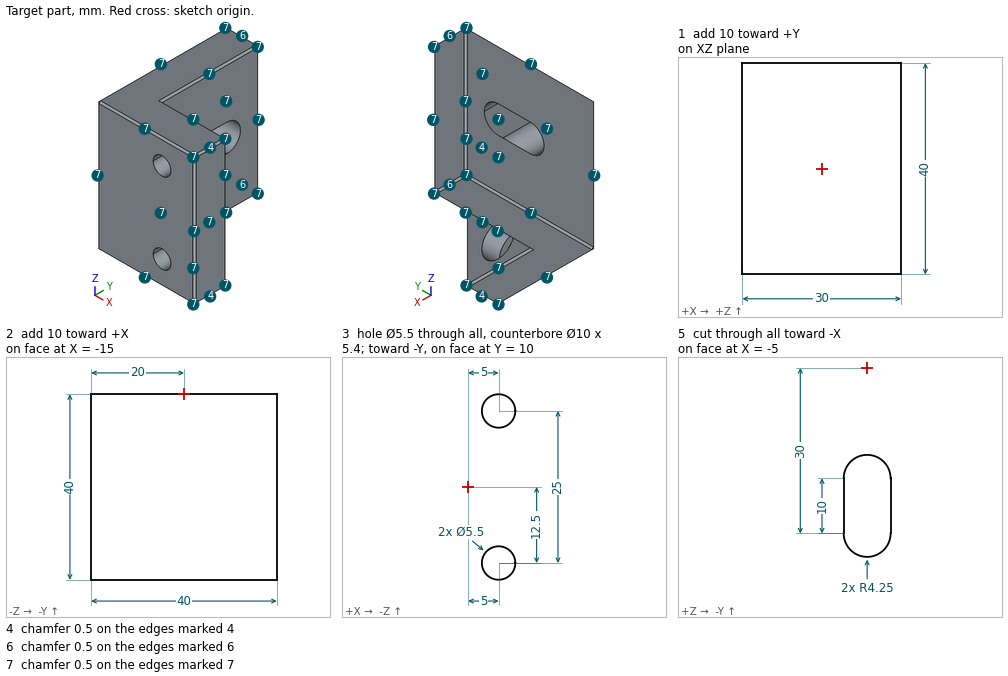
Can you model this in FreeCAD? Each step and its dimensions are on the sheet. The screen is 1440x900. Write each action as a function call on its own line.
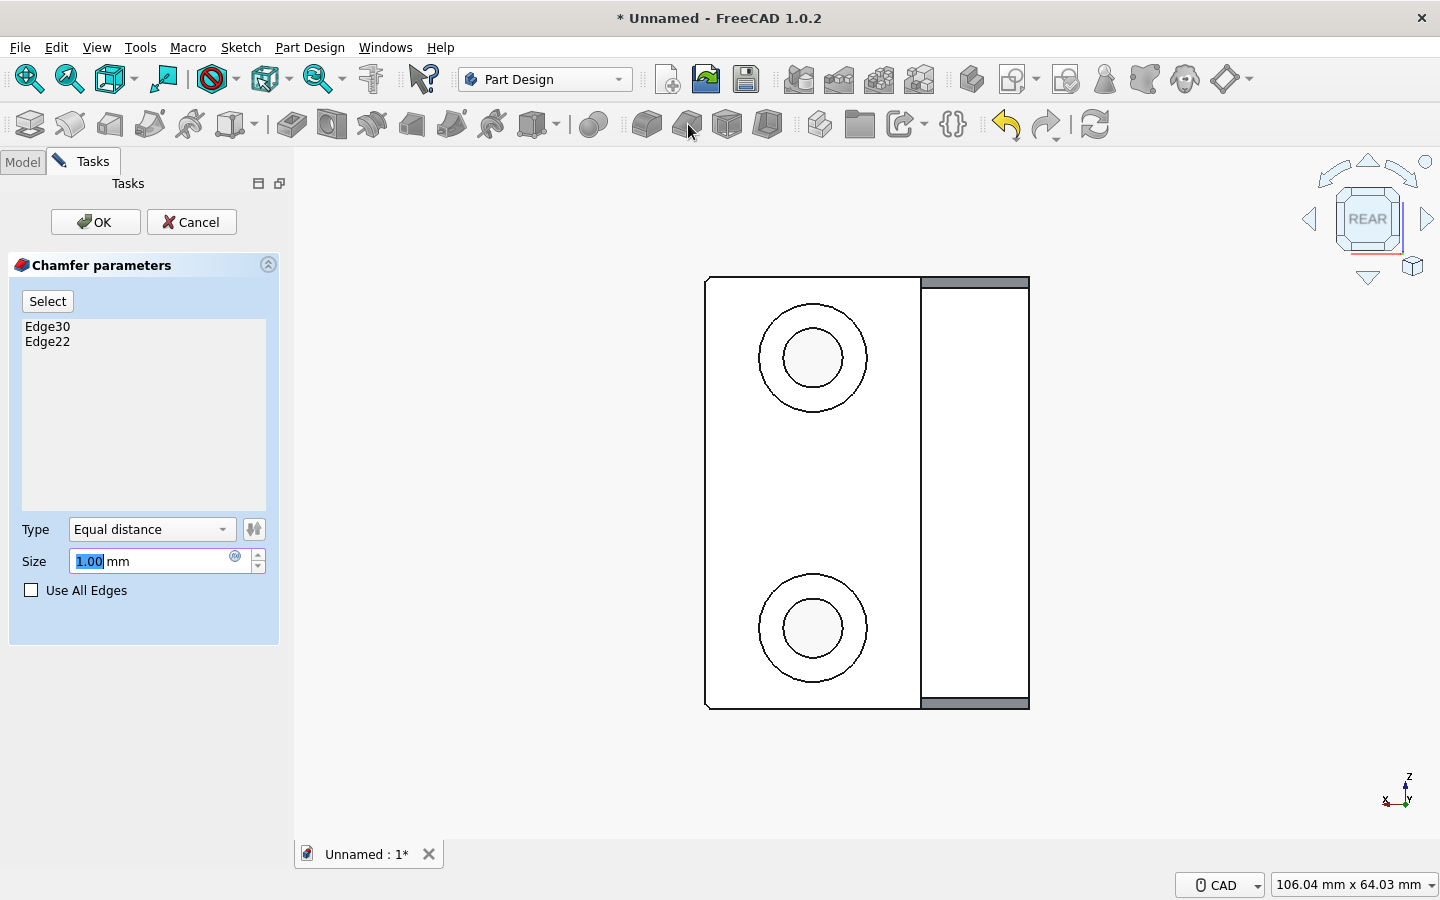
text(0.5)
key(Tab)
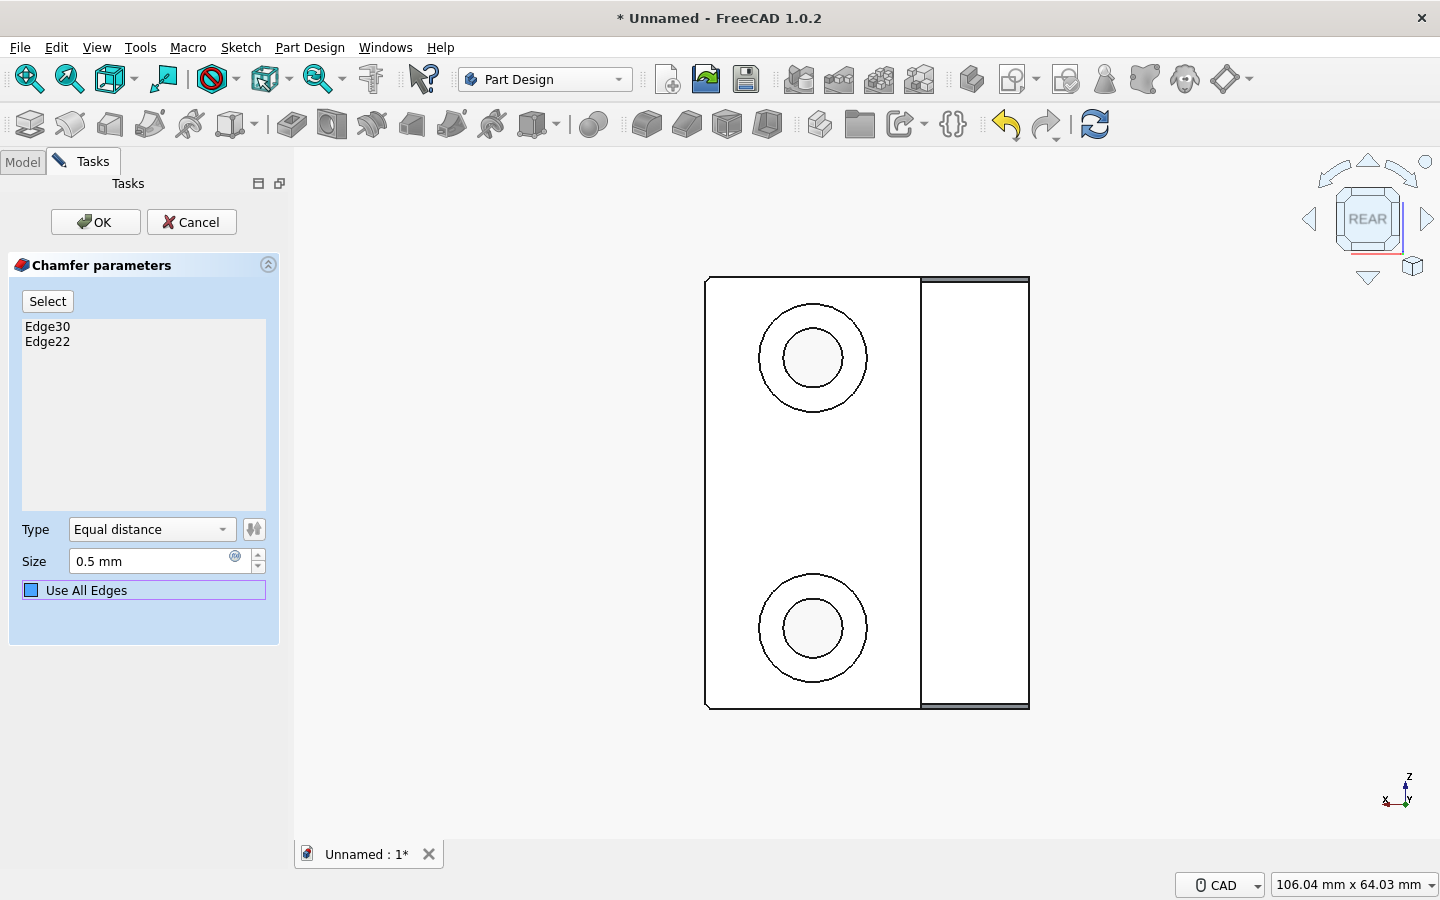
click(96, 222)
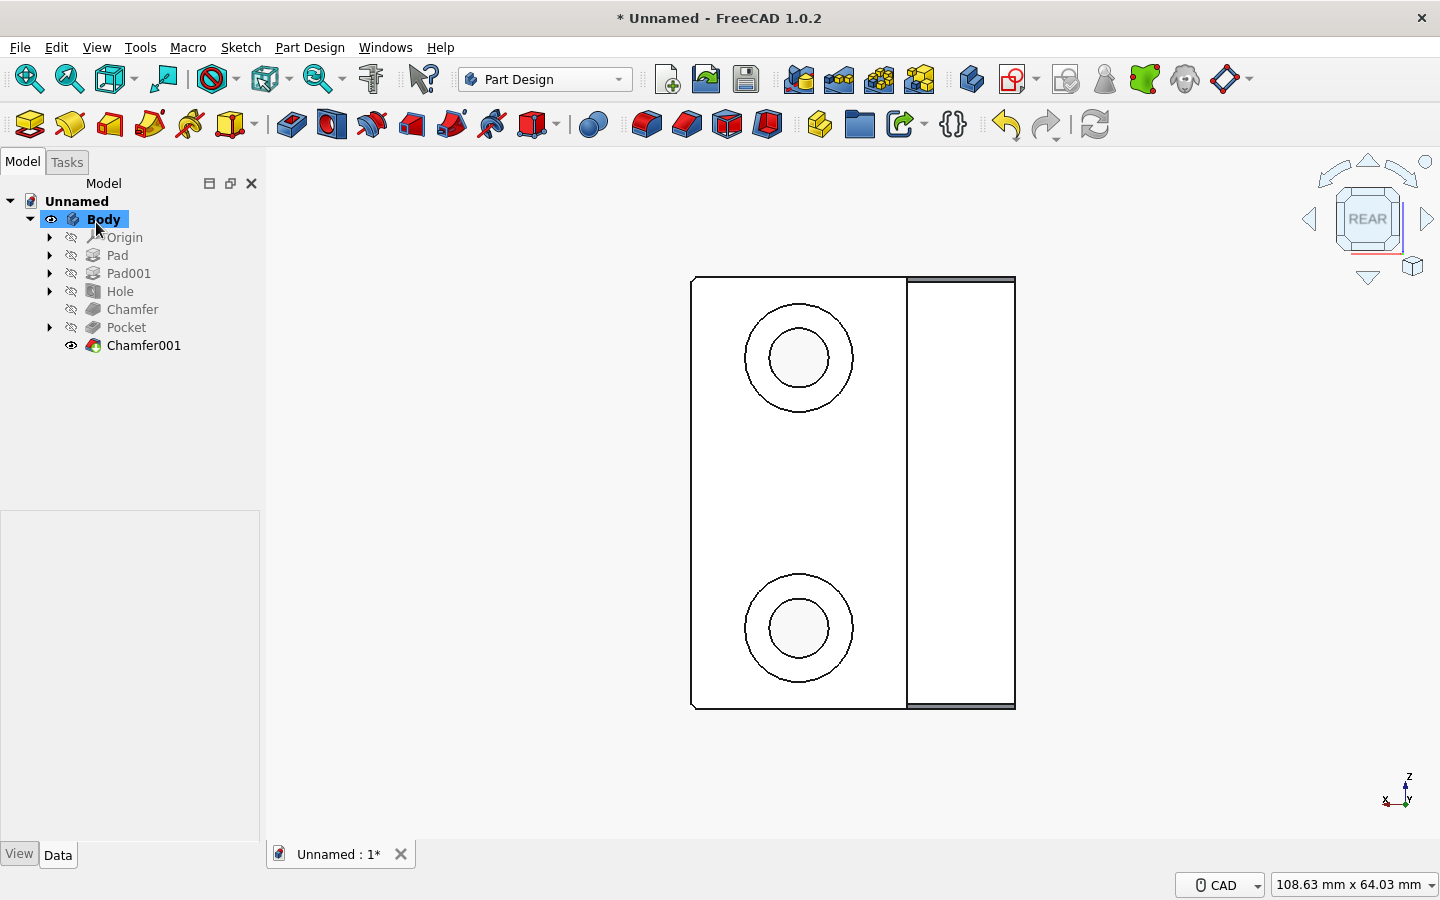
click(802, 708)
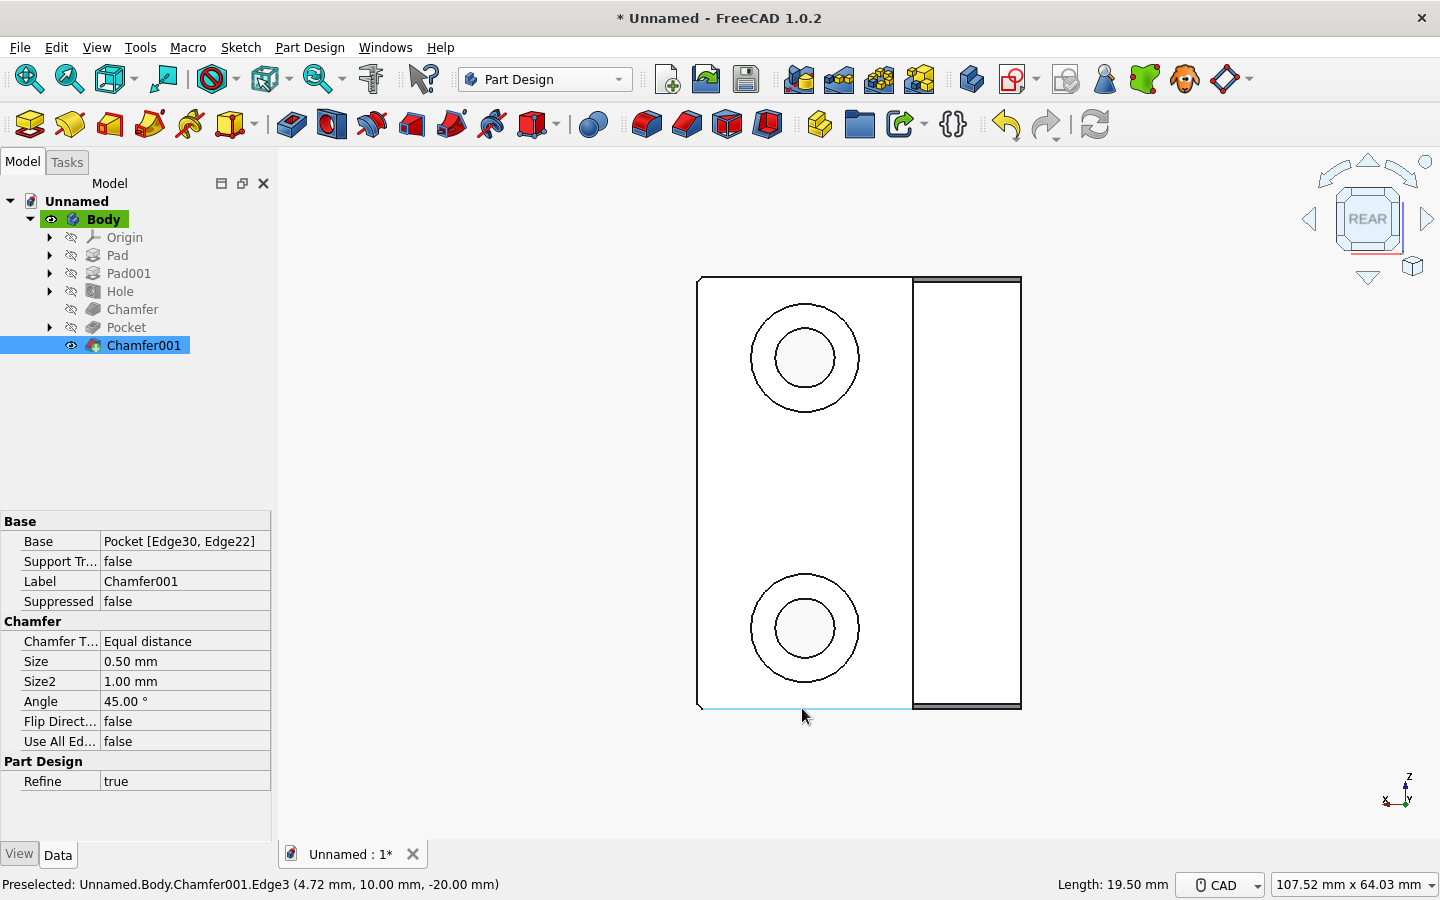
click(697, 492, ctrl)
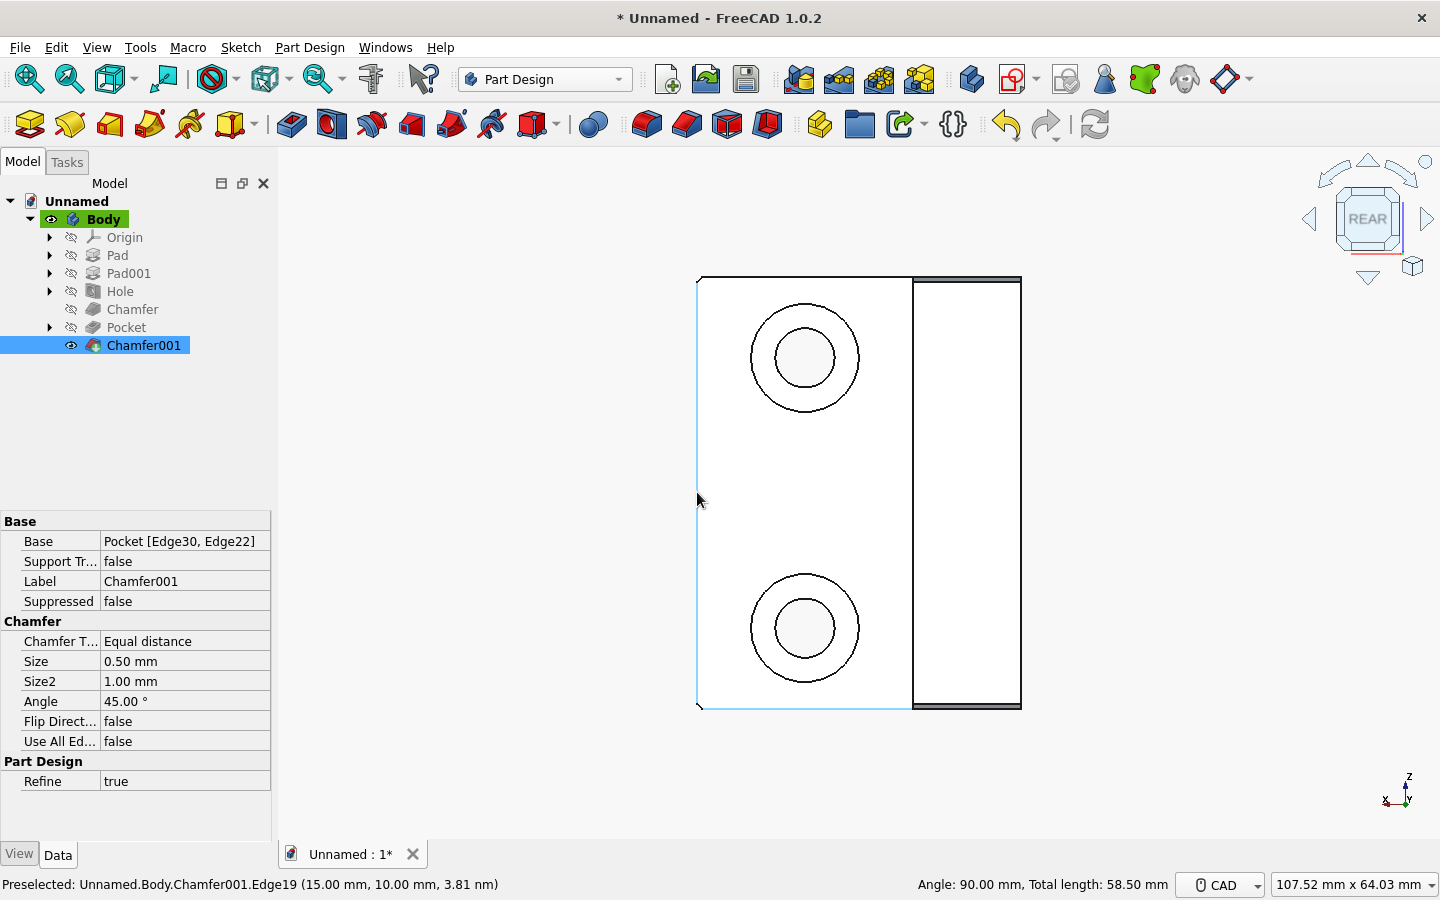
click(1021, 492, ctrl)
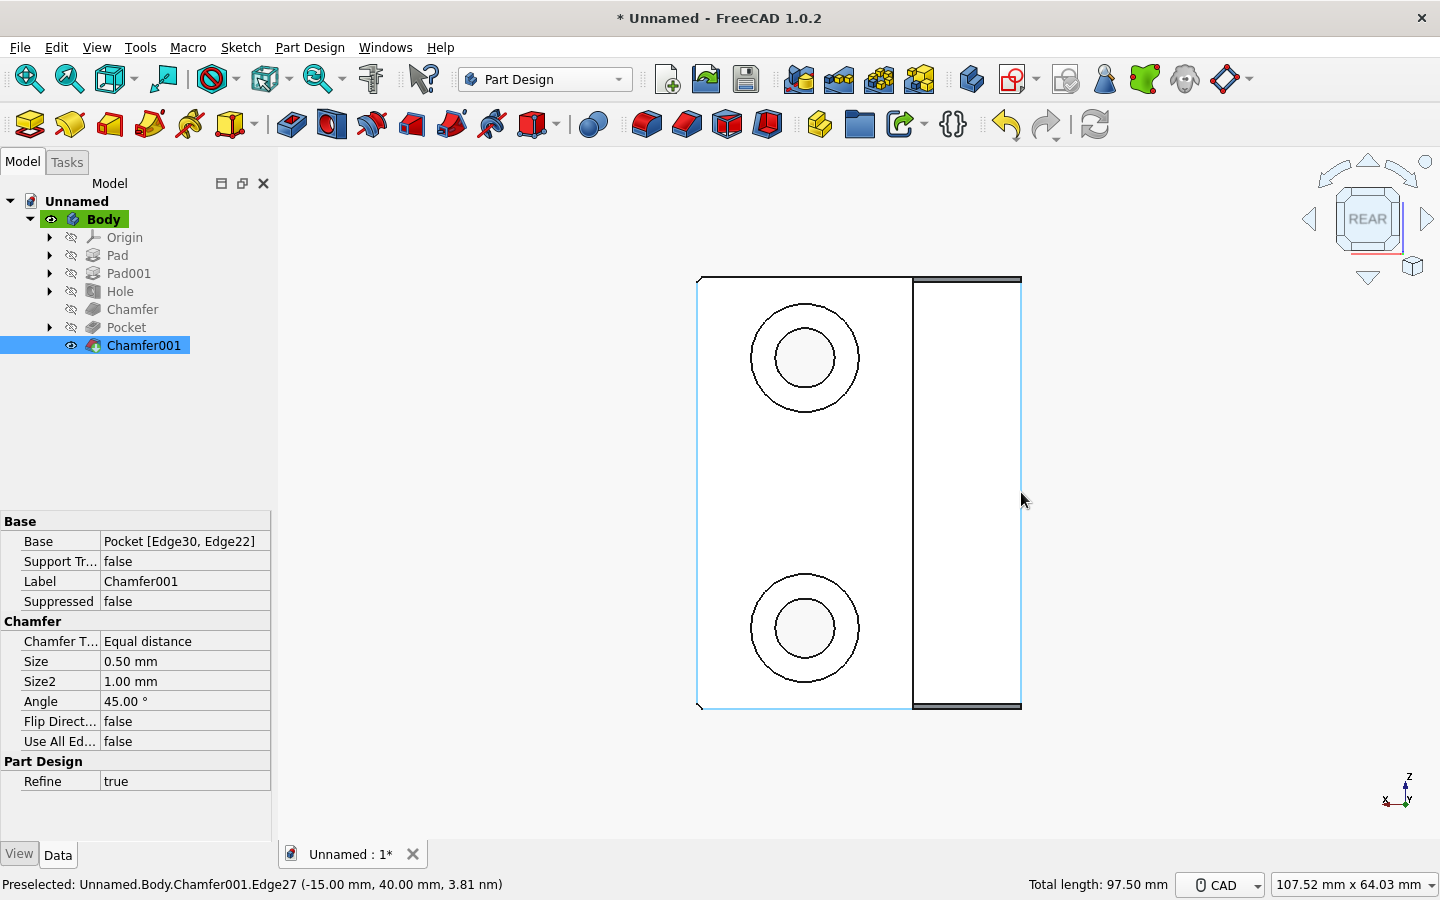
click(913, 492, ctrl)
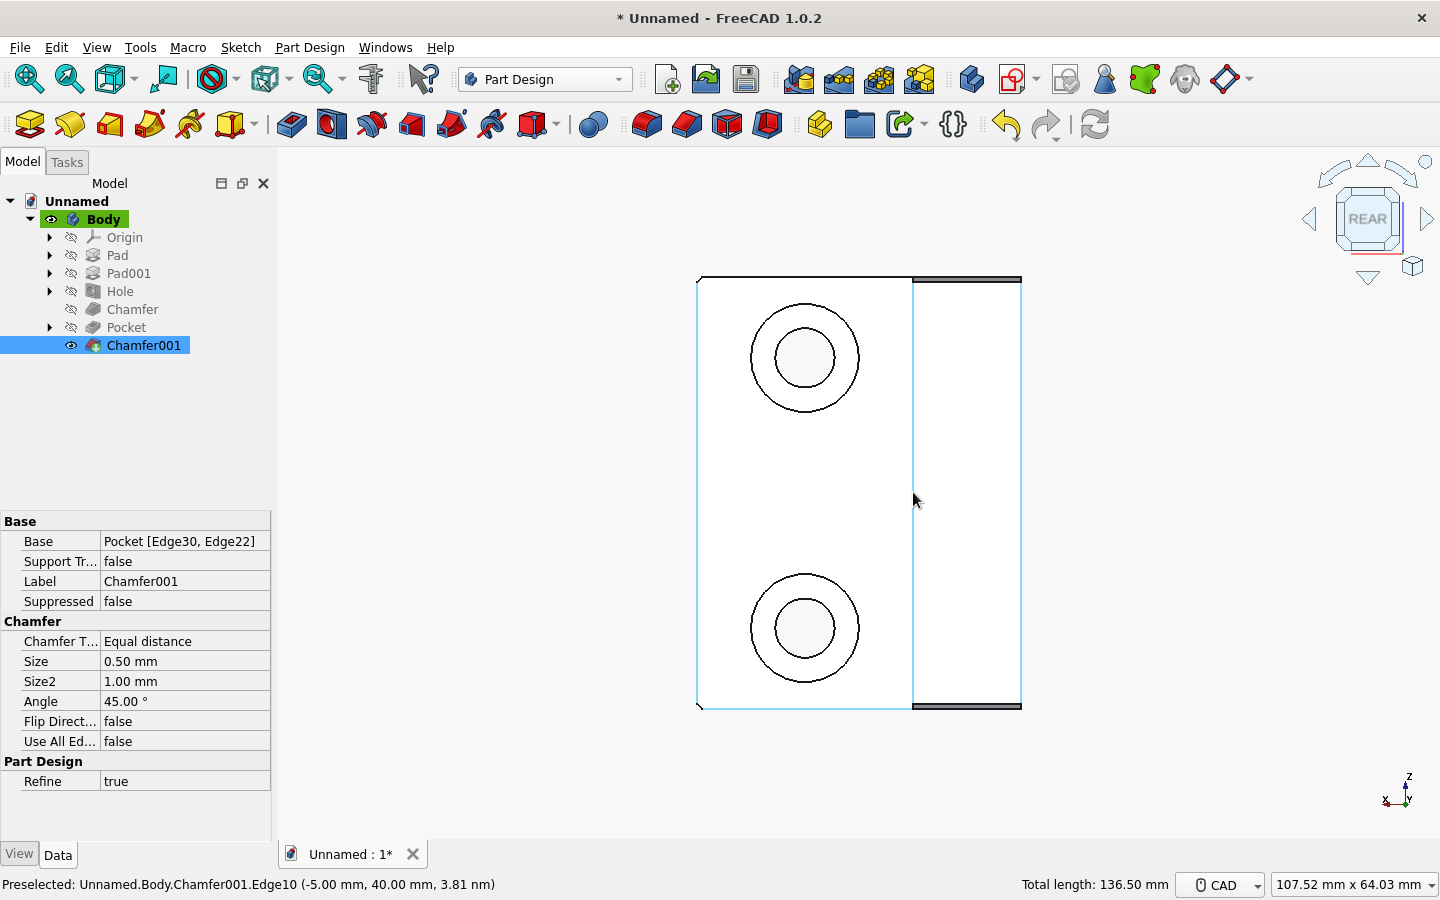
key(0)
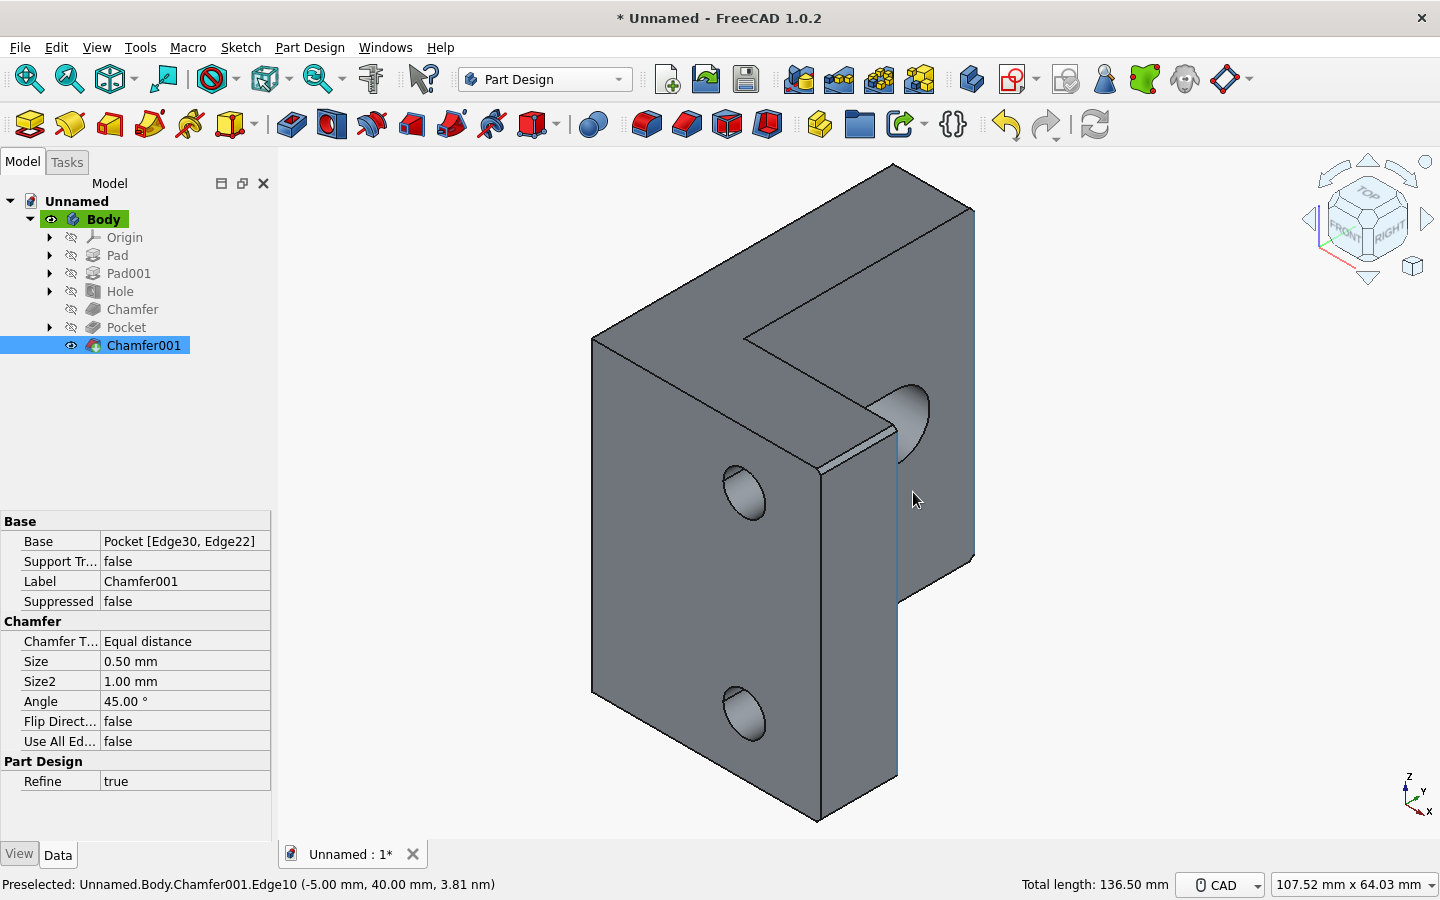
click(857, 273, ctrl)